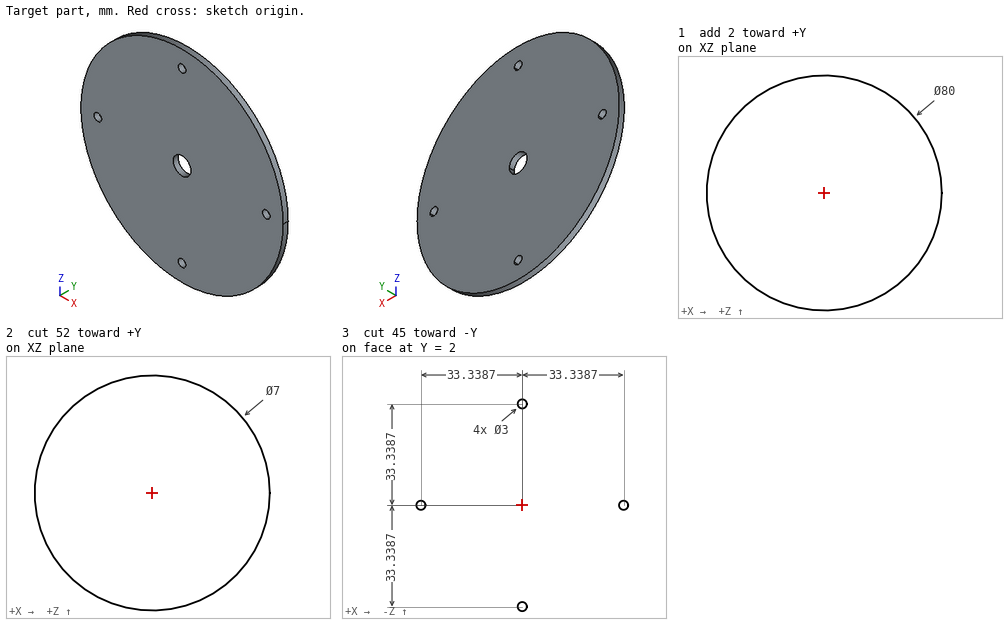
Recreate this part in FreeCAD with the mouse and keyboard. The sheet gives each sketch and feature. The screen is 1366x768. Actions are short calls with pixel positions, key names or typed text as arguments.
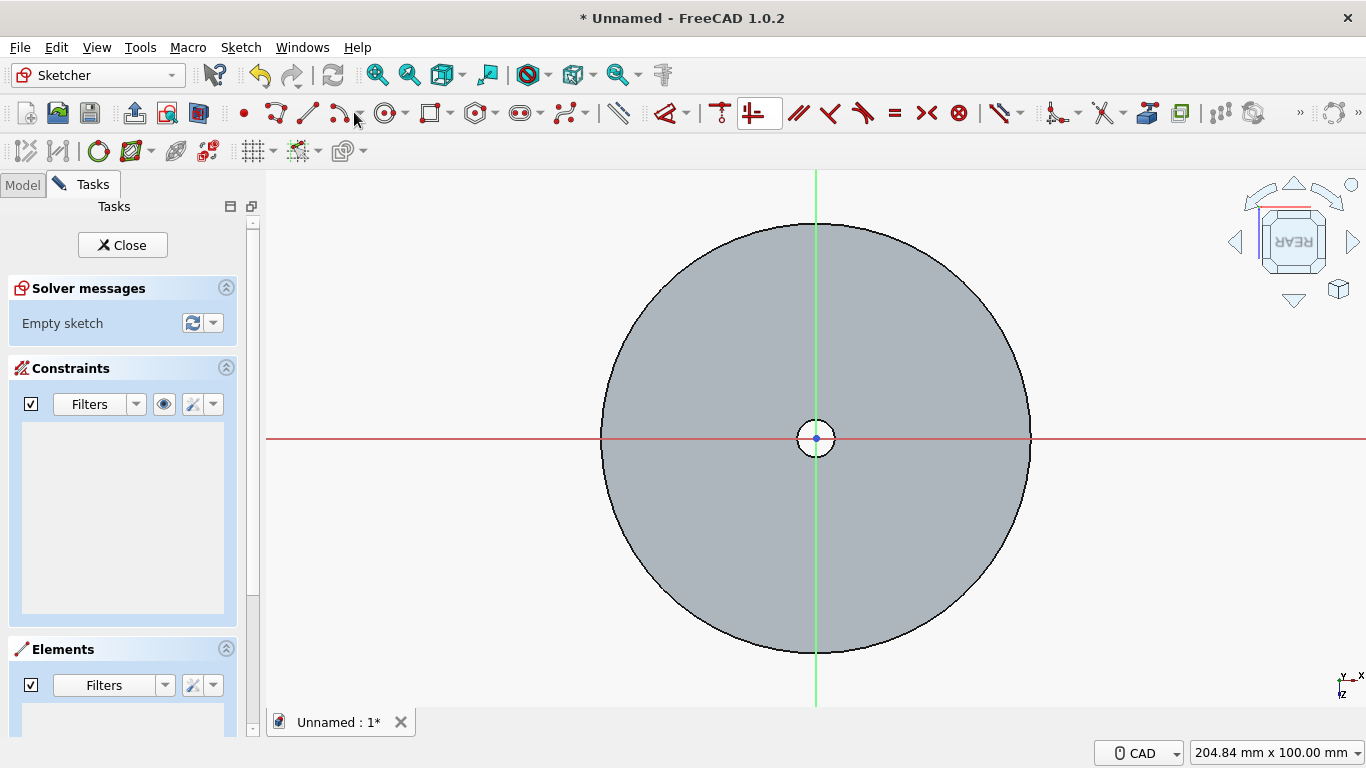
key(g)
key(c)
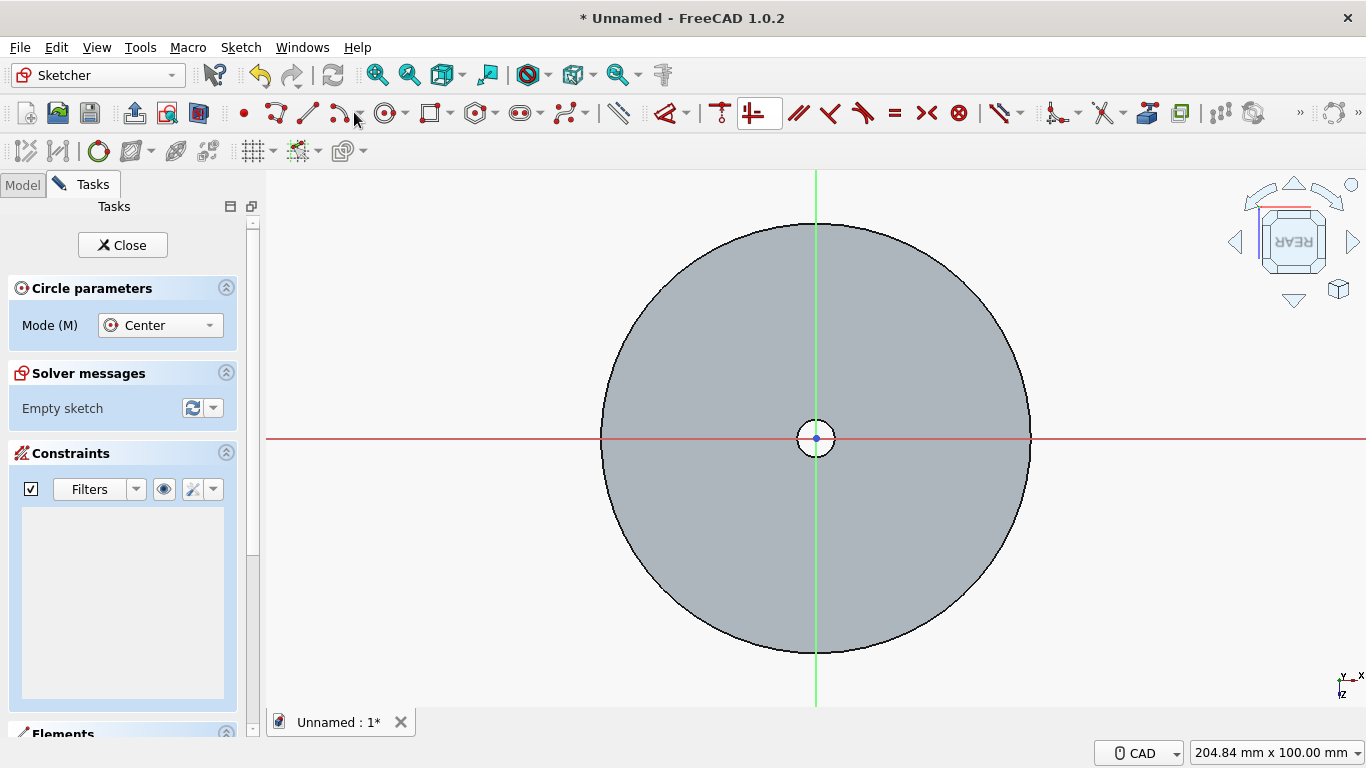
scroll(816, 259, up, 6)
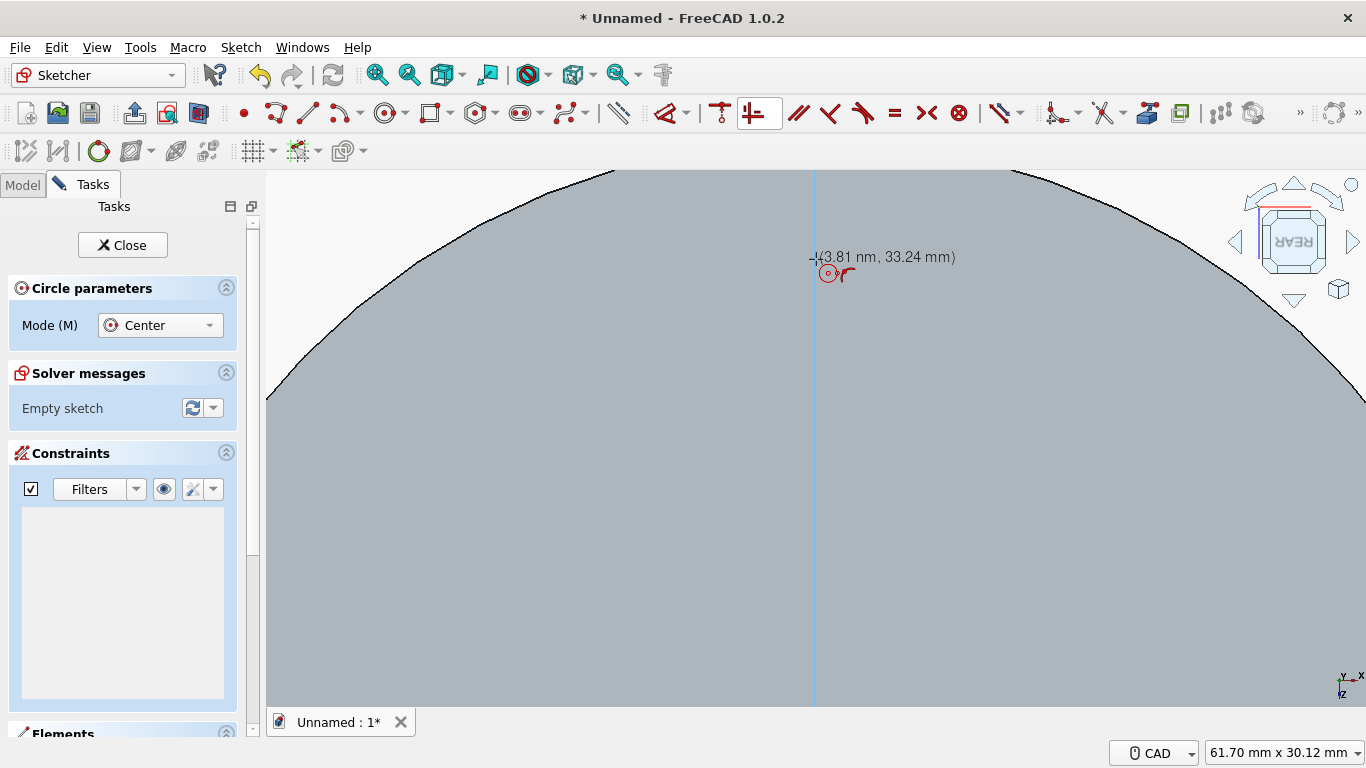
click(815, 260)
click(834, 241)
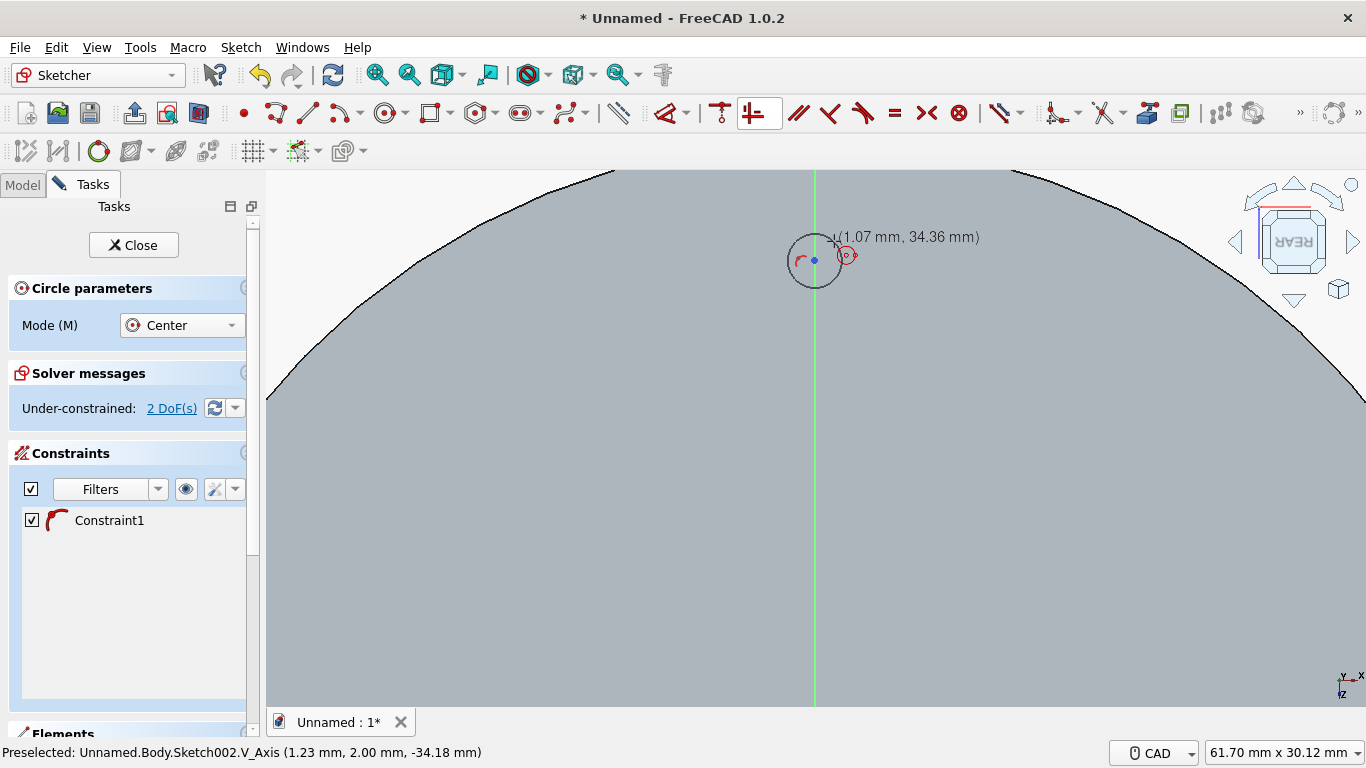
scroll(718, 259, down, 6)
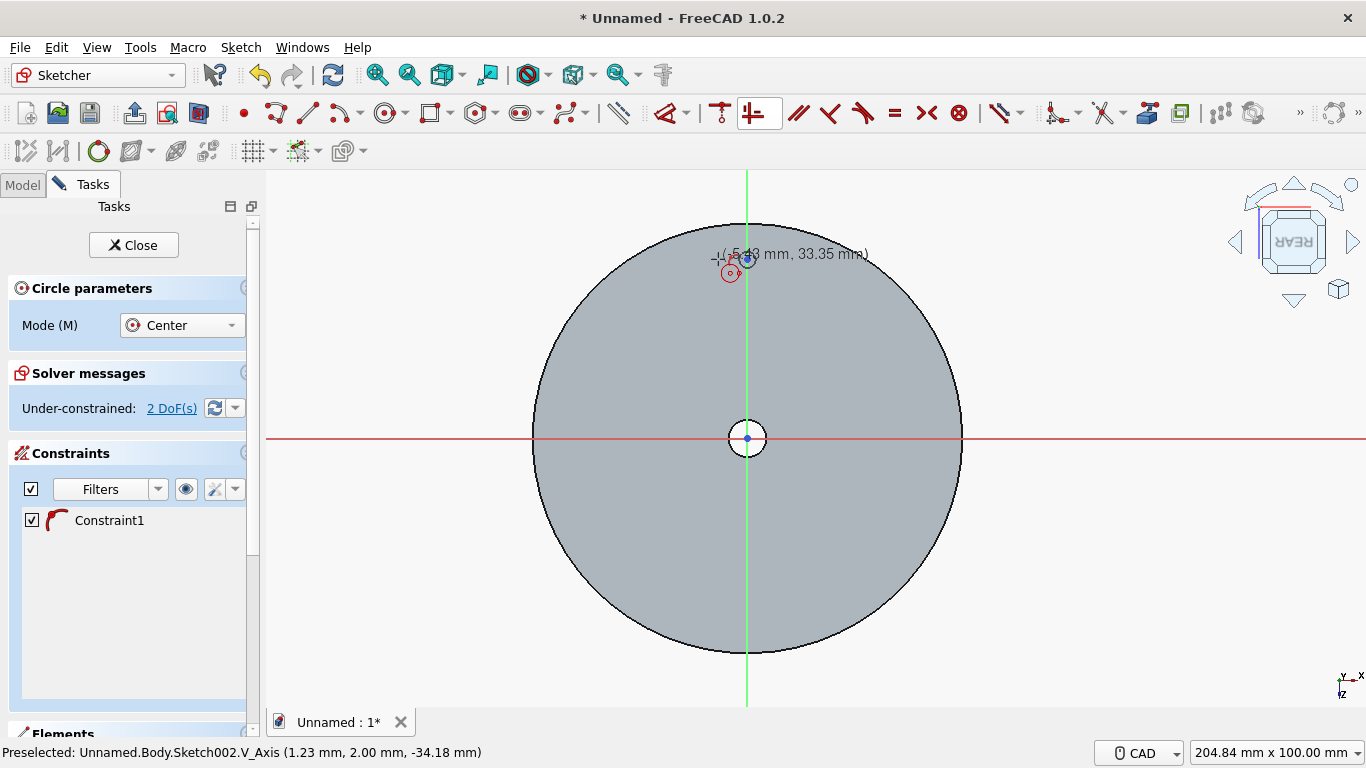
scroll(926, 438, up, 6)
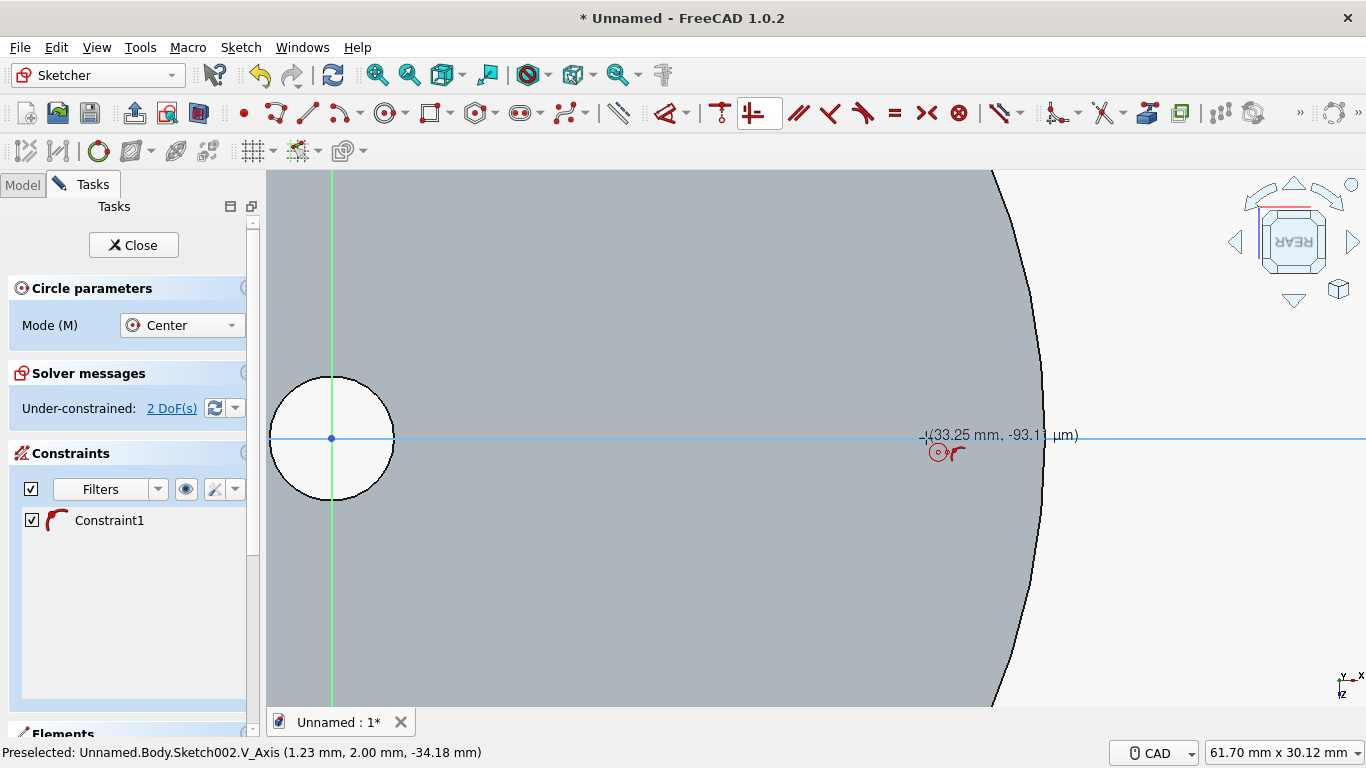
click(926, 438)
click(945, 420)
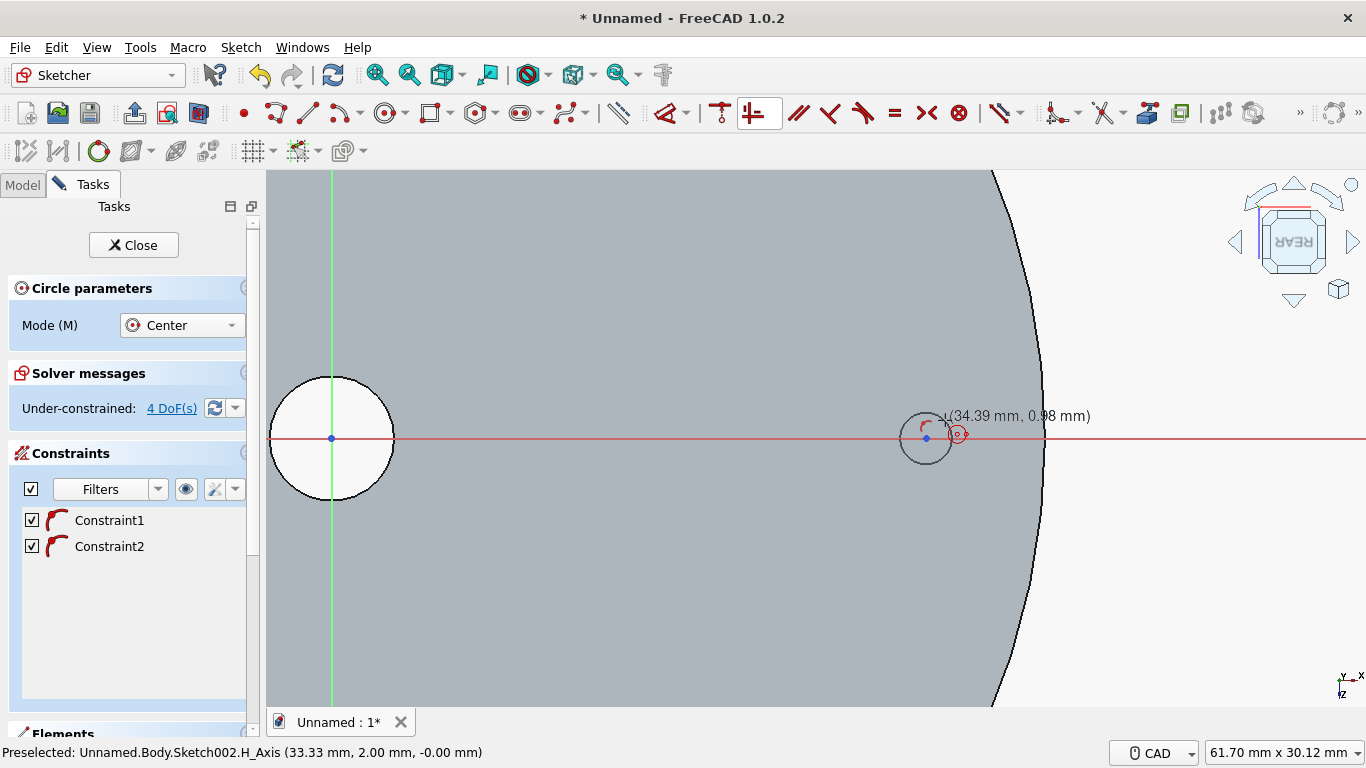
scroll(927, 438, down, 6)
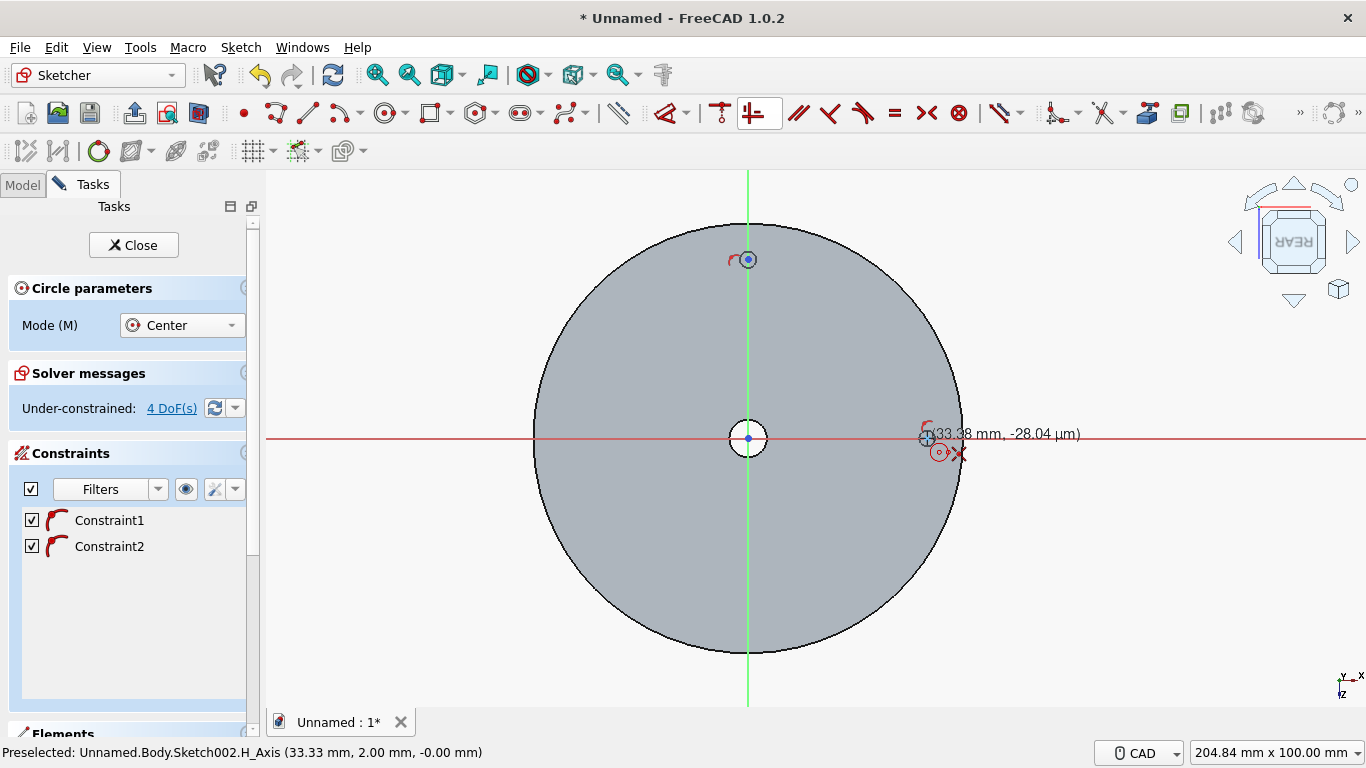
scroll(748, 618, up, 6)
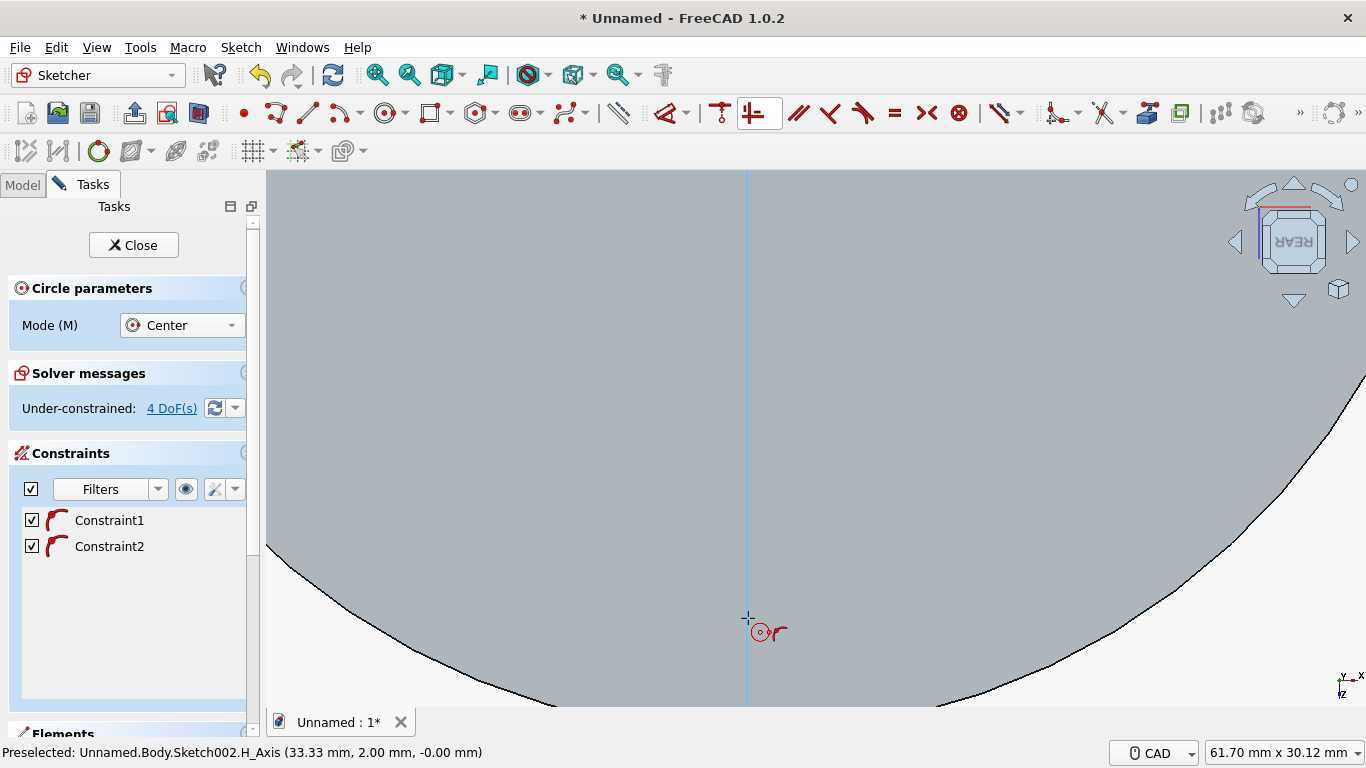
click(747, 614)
click(766, 596)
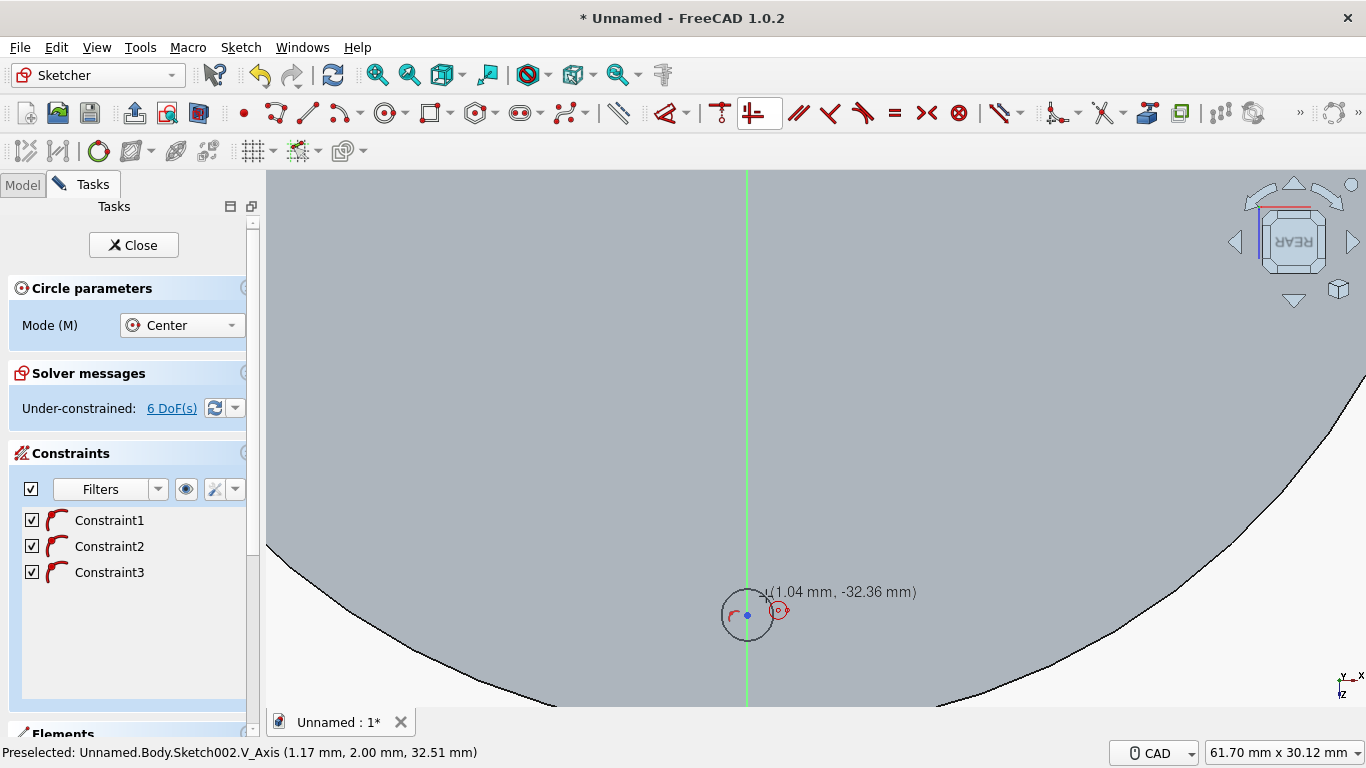
scroll(748, 619, down, 6)